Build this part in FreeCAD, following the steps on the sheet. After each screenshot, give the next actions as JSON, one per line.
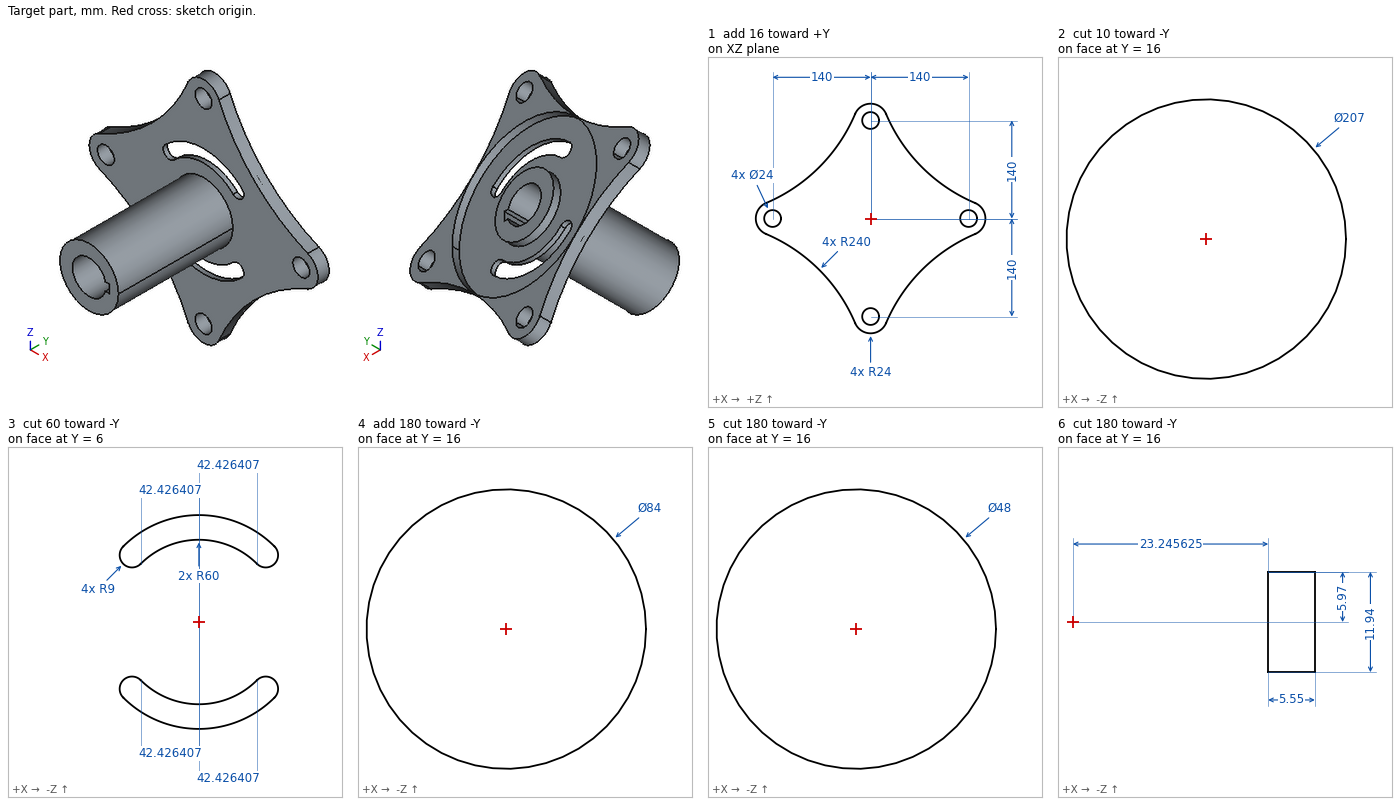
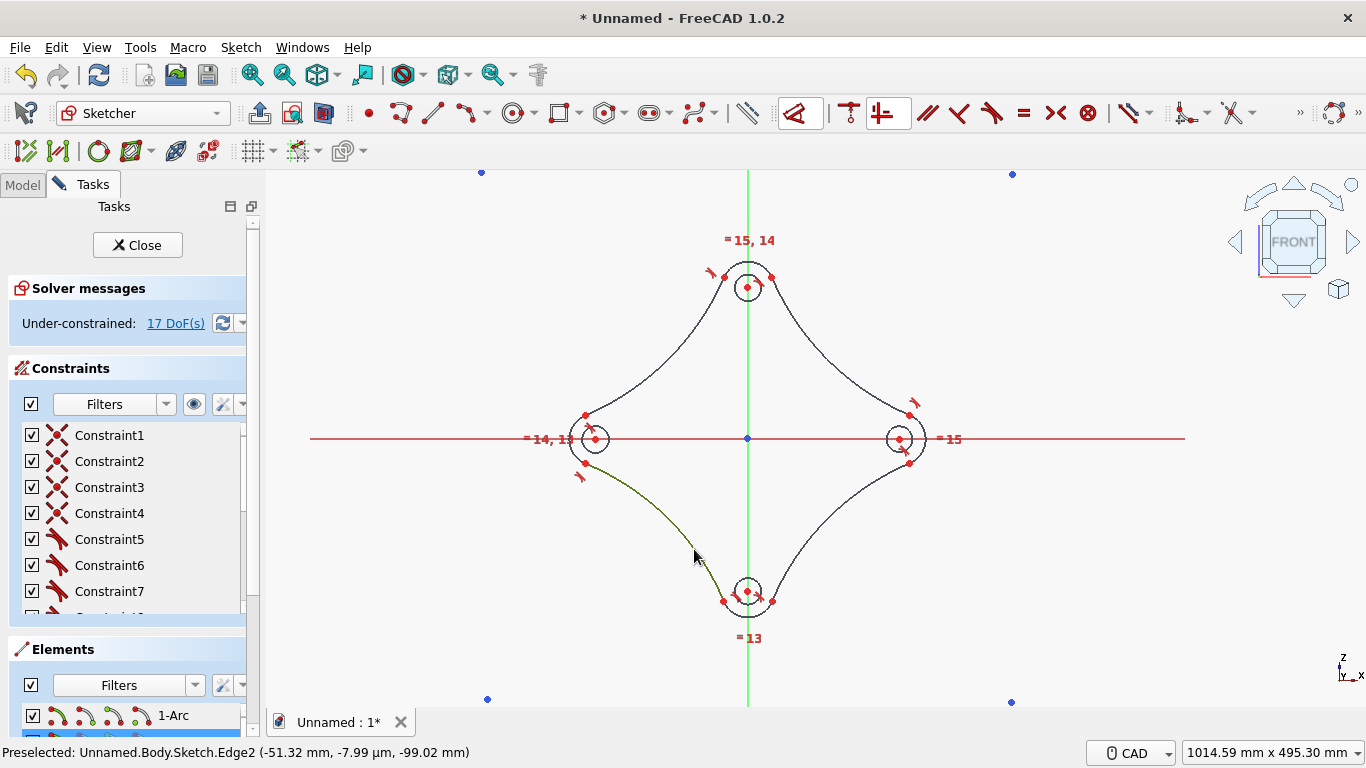
{"action": "left_click", "coordinate": [637, 386]}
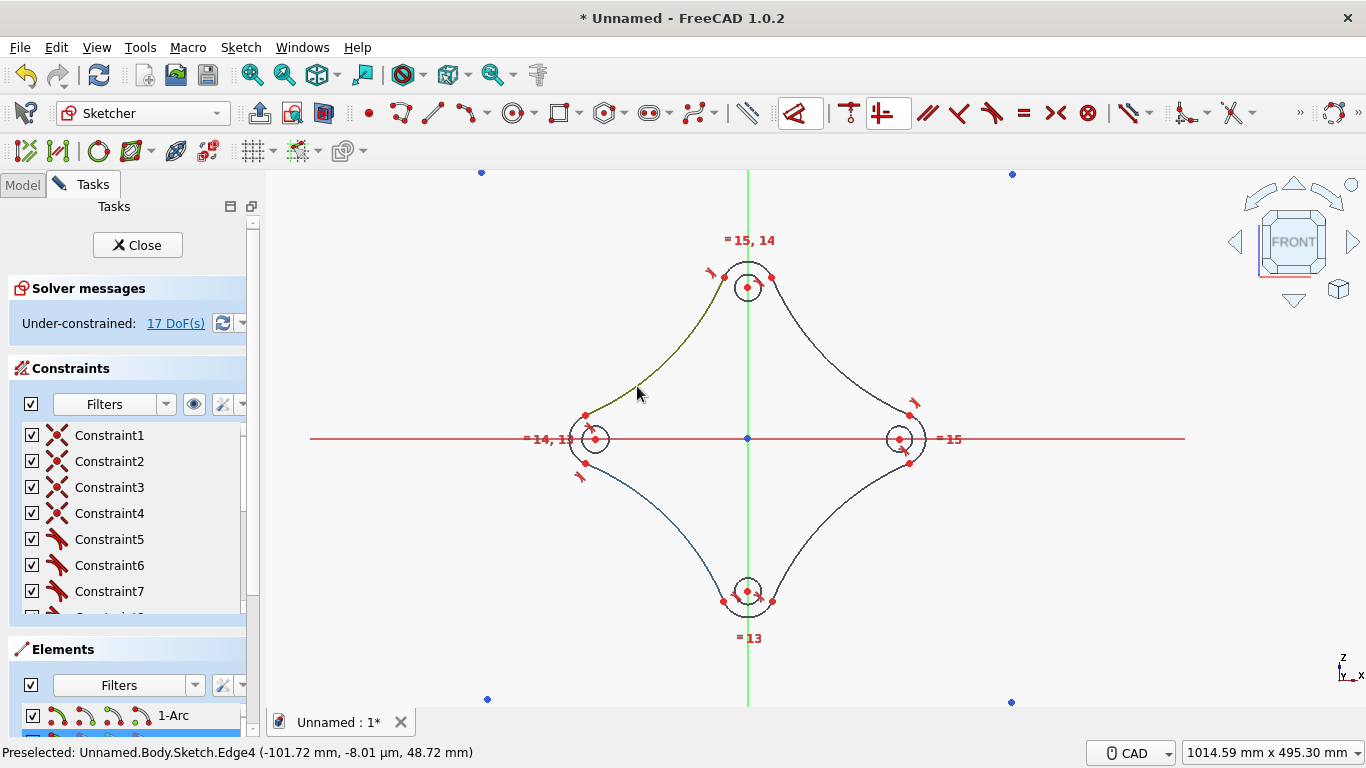
{"action": "left_click", "coordinate": [802, 329]}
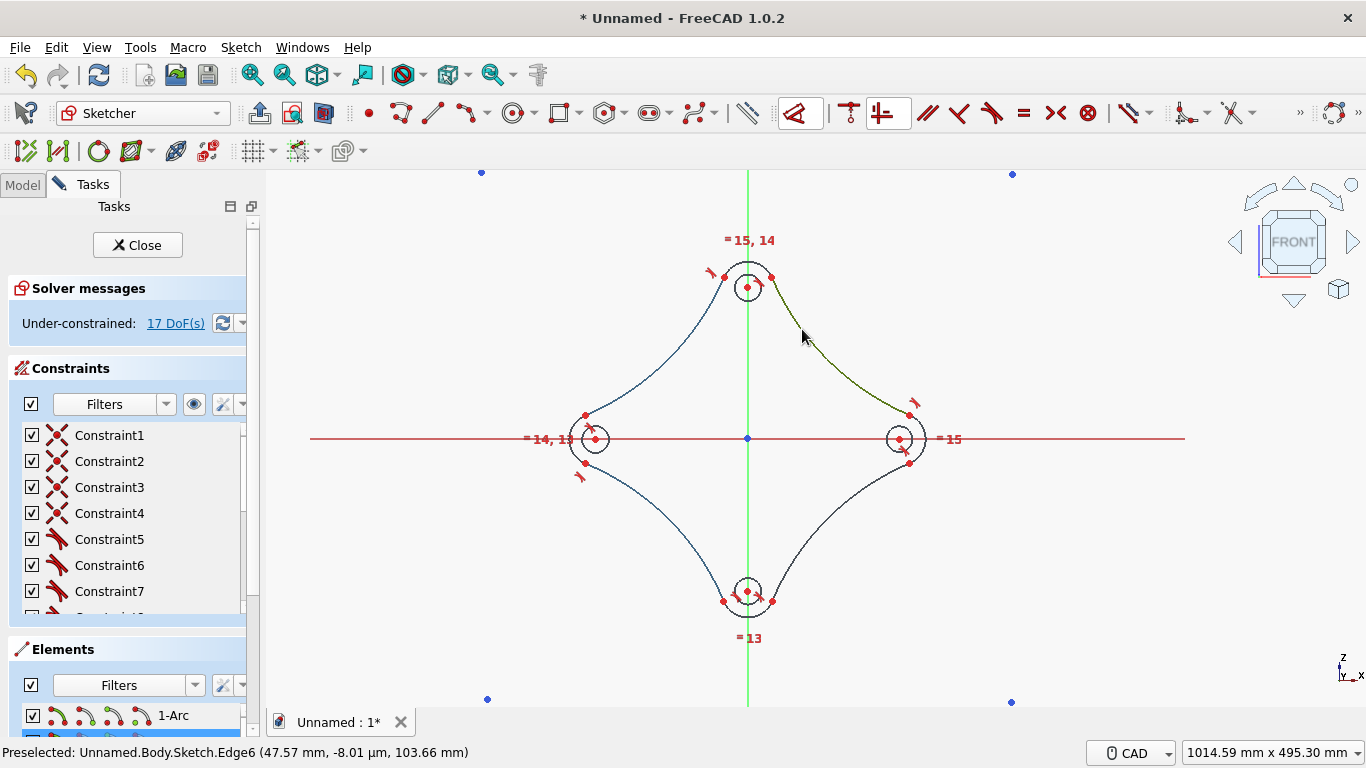
{"action": "left_click", "coordinate": [858, 493]}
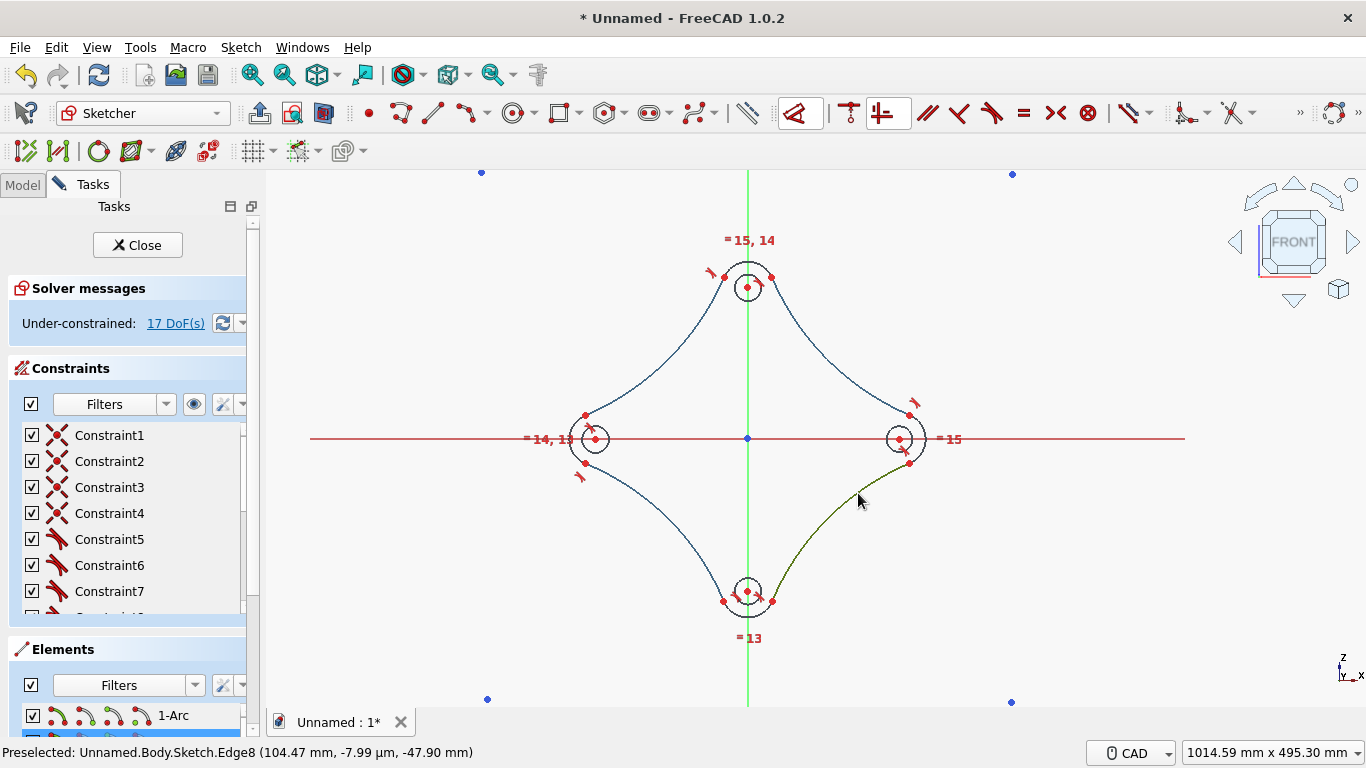
{"action": "left_click", "coordinate": [1024, 114]}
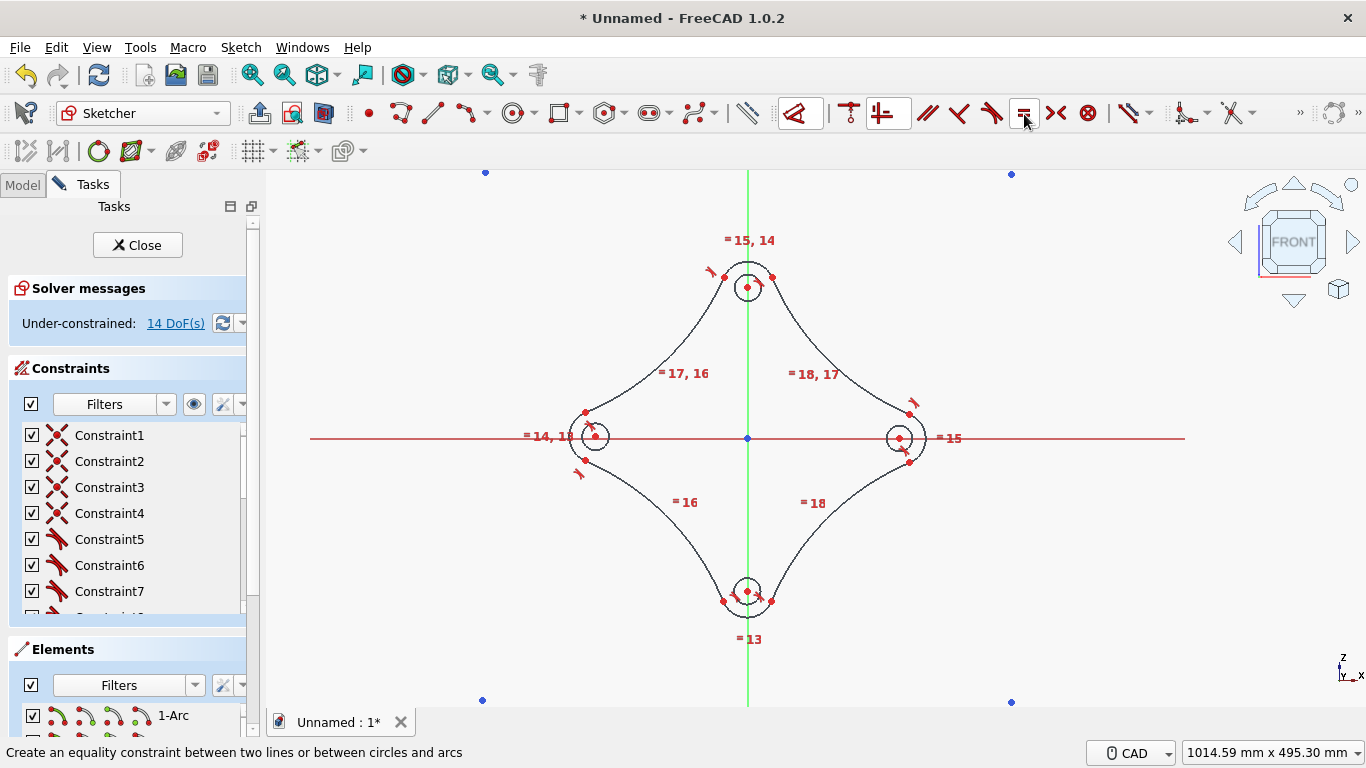
{"action": "scroll", "coordinate": [757, 279], "scroll_direction": "up", "scroll_amount": 2}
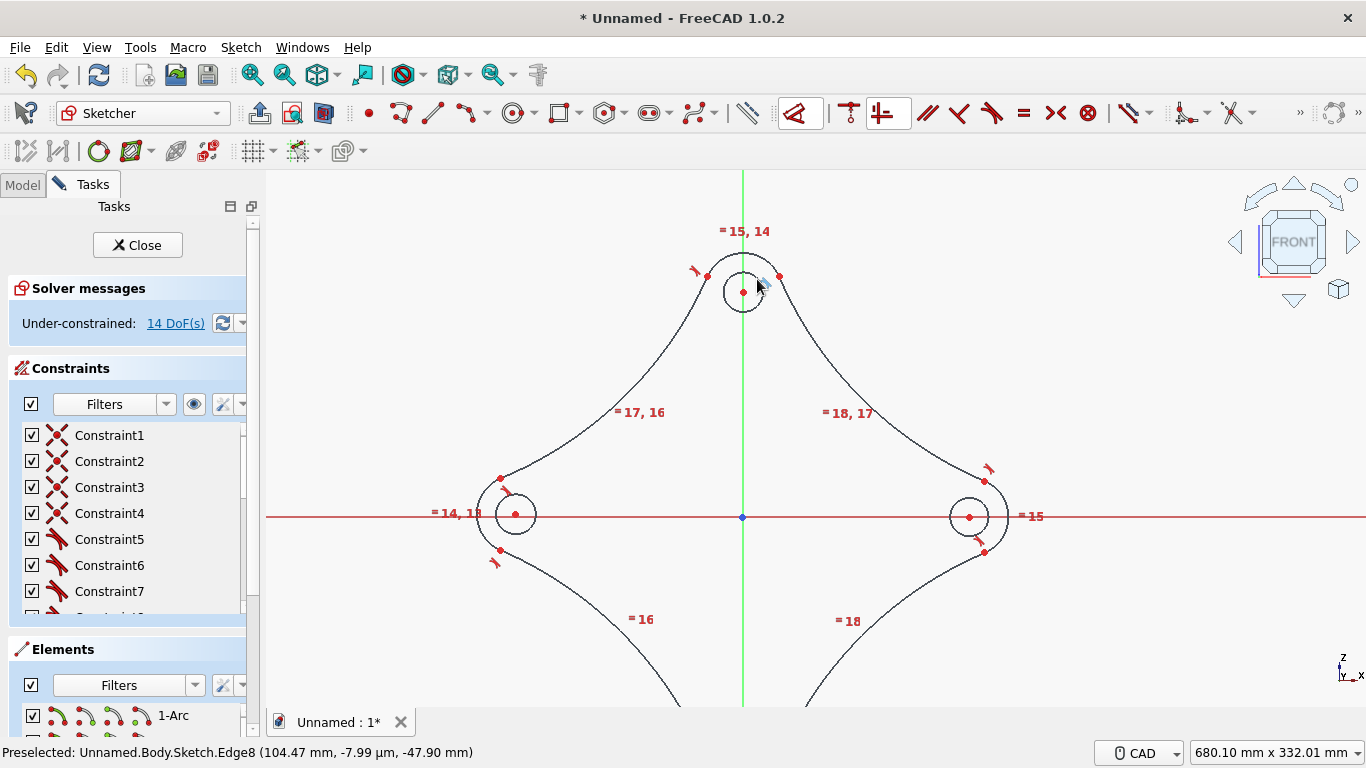
{"action": "left_click", "coordinate": [757, 278]}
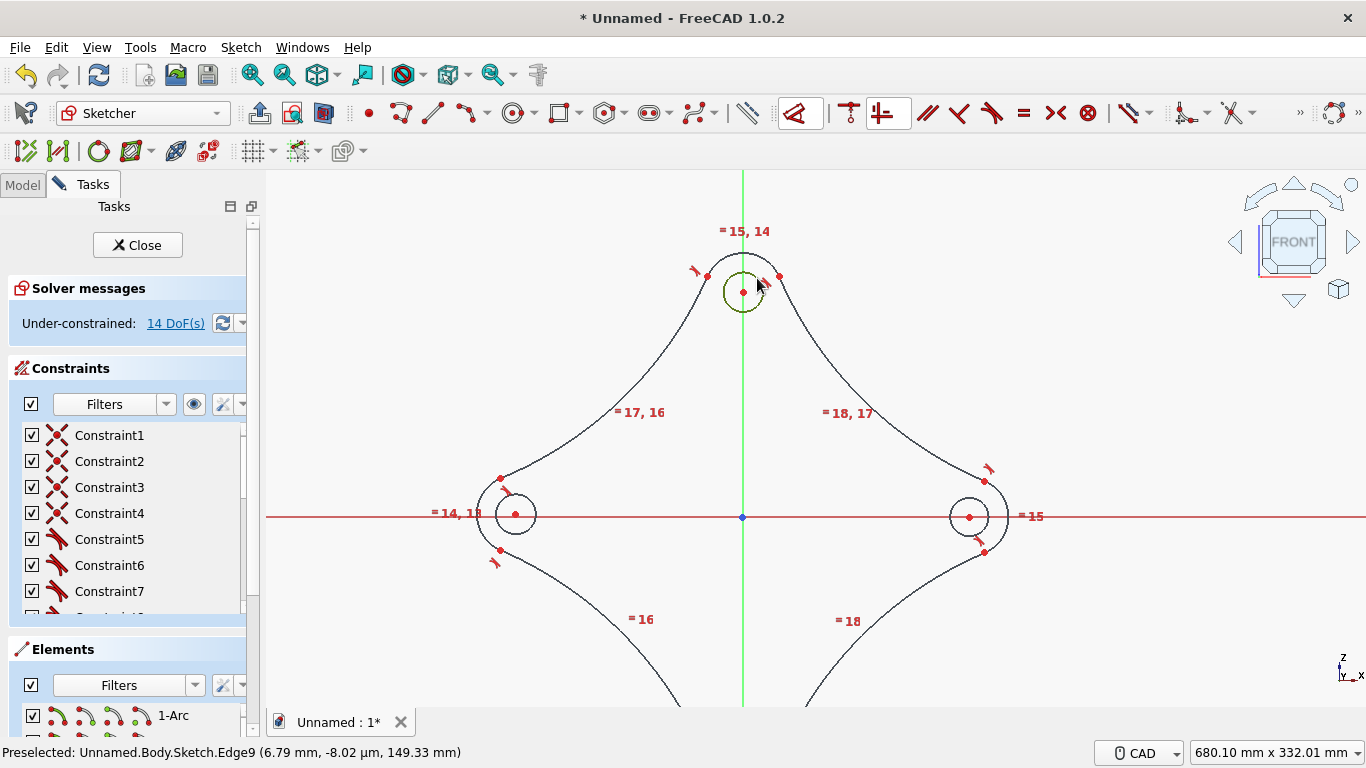
{"action": "left_click", "coordinate": [530, 500]}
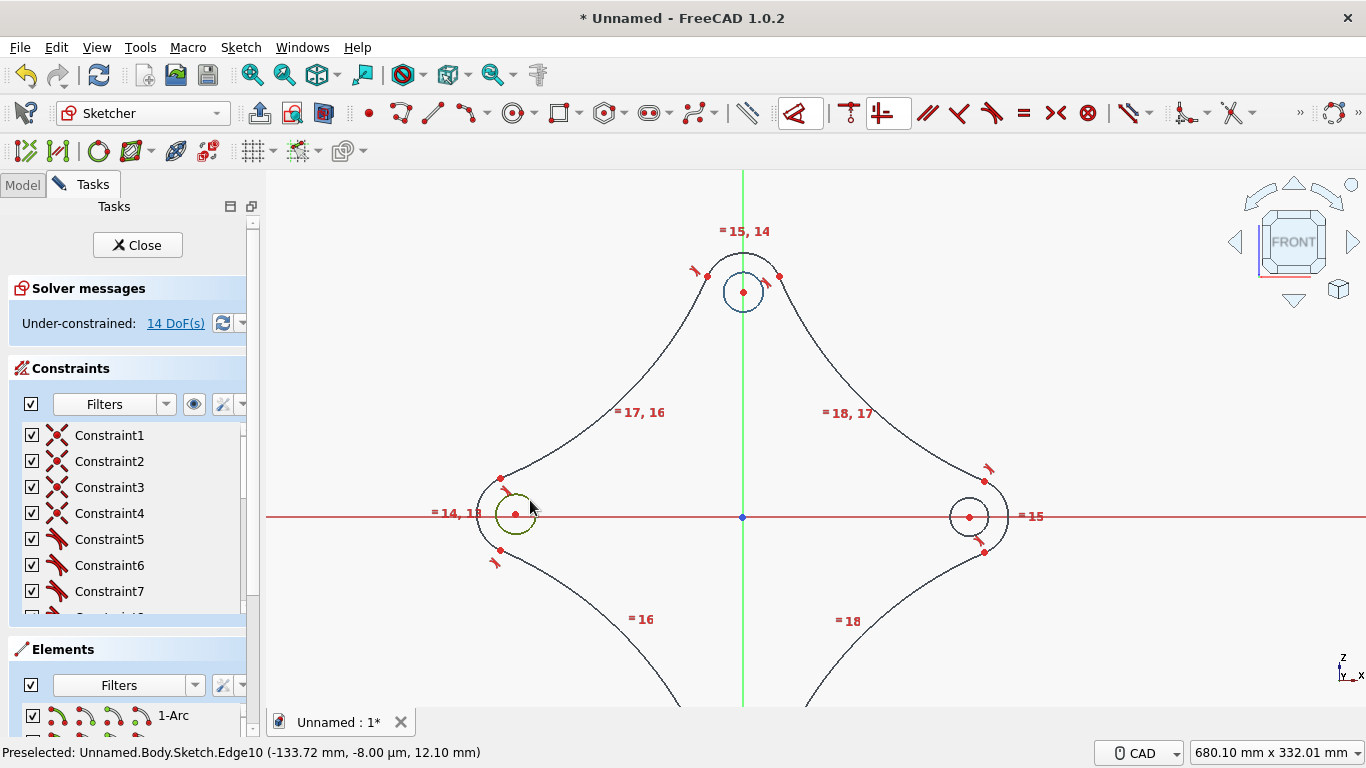
{"action": "left_click", "coordinate": [983, 503]}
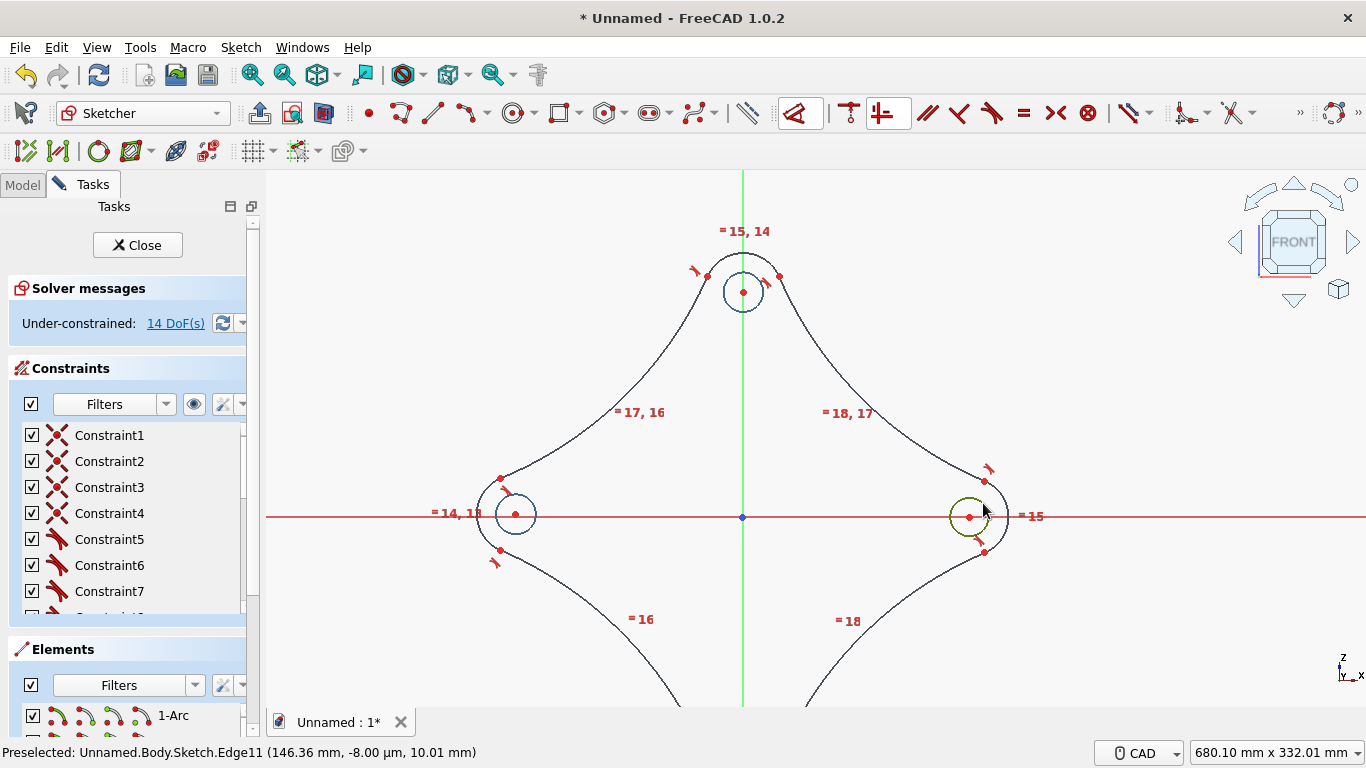
{"action": "scroll", "coordinate": [757, 279], "scroll_direction": "down", "scroll_amount": 2}